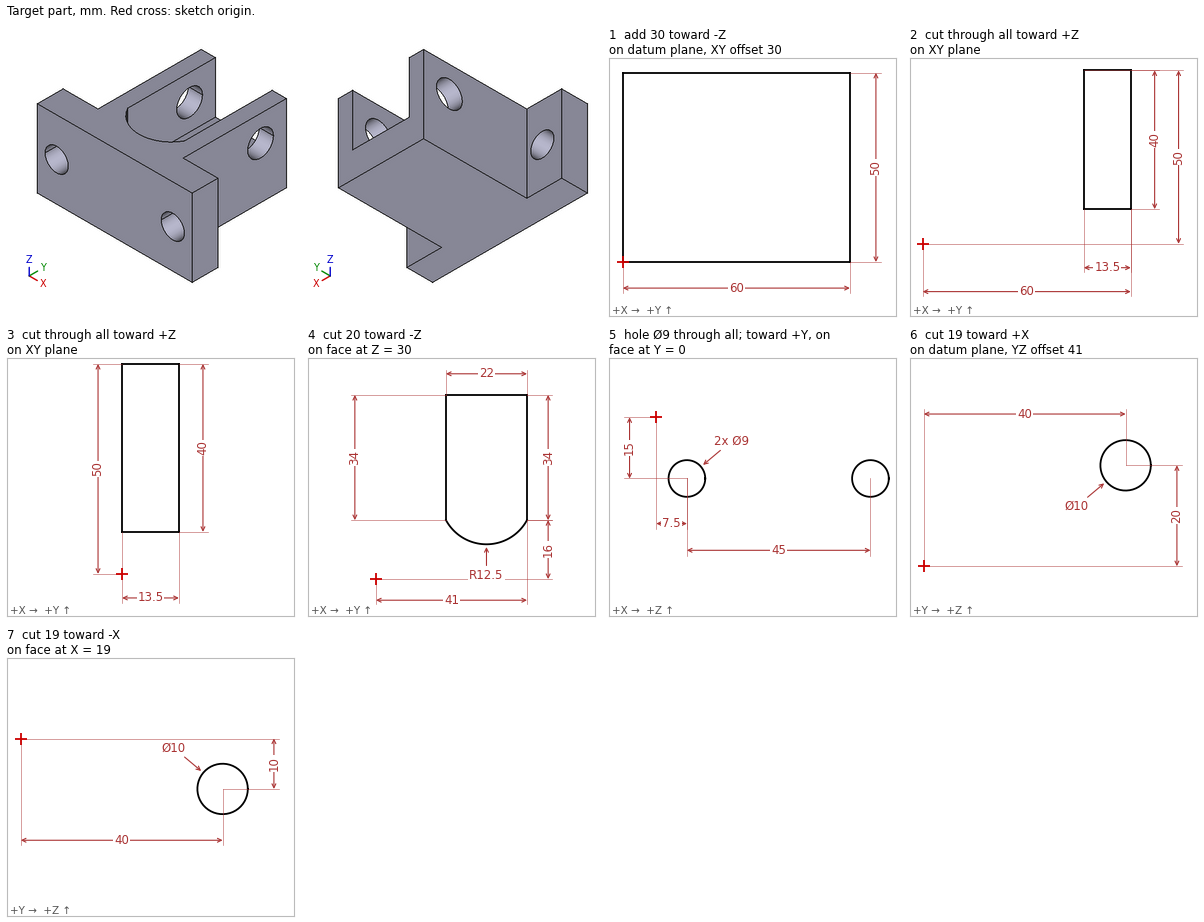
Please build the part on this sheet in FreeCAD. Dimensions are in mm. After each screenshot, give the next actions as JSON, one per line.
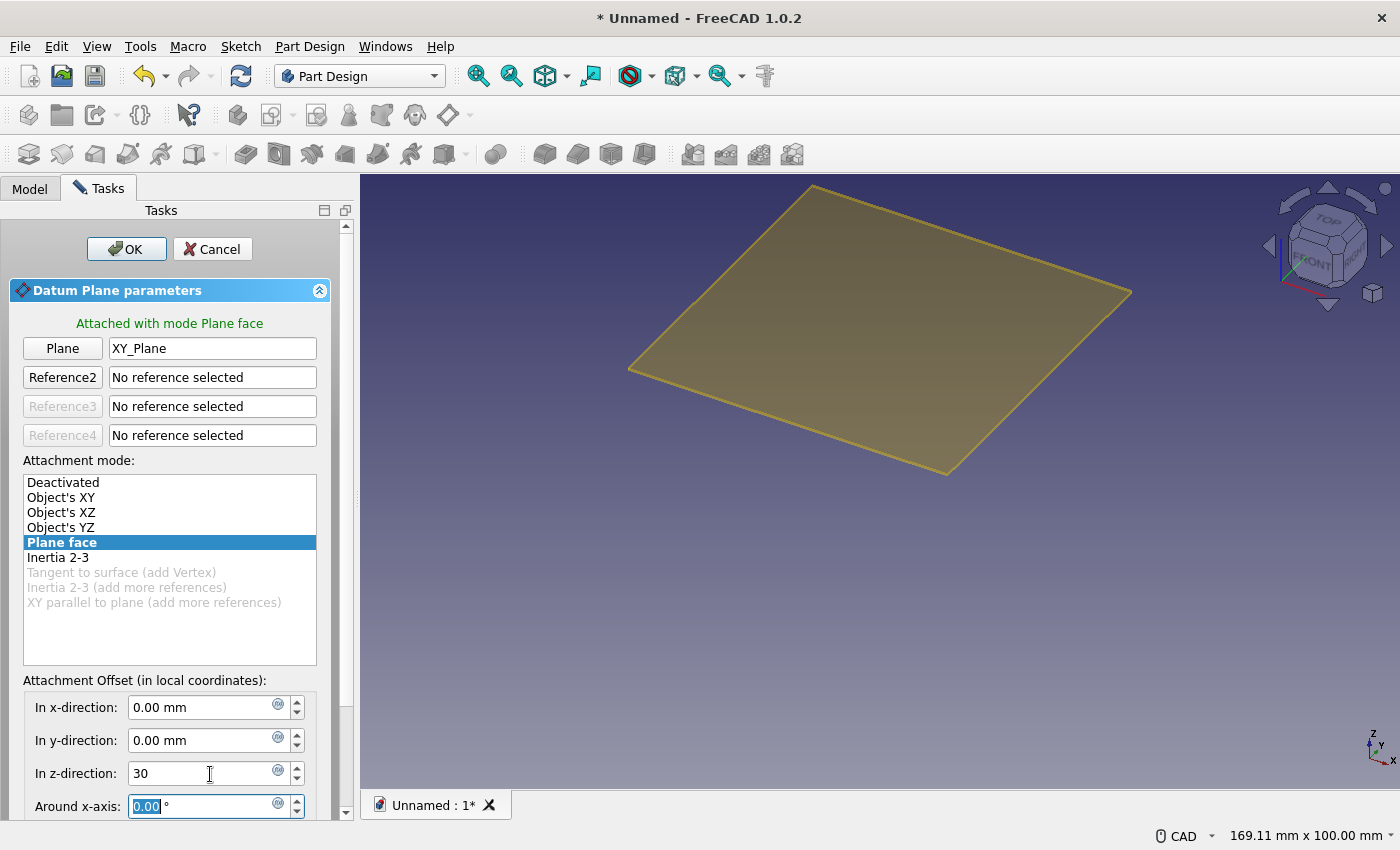
{"action": "left_click", "coordinate": [127, 249]}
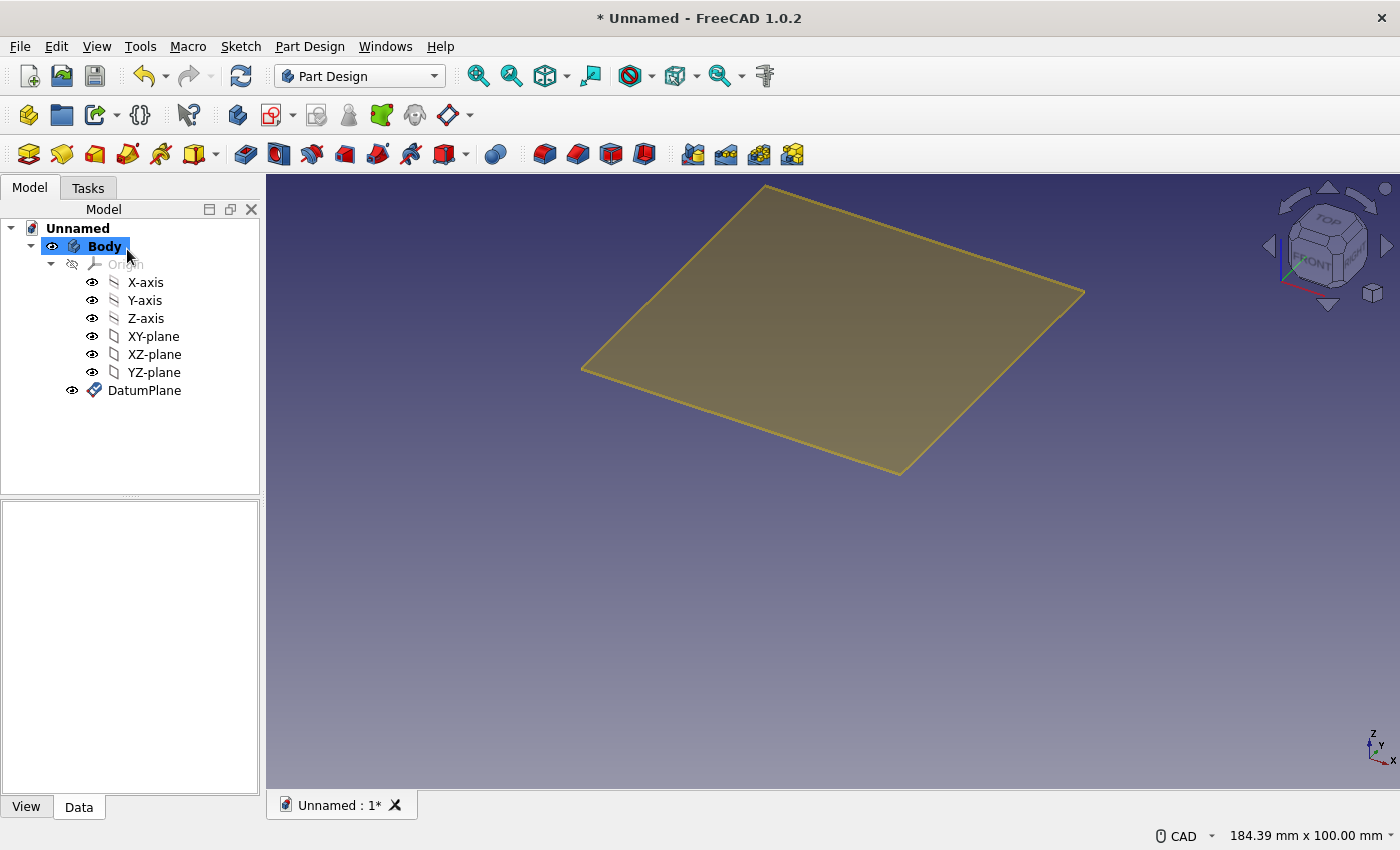
{"action": "left_click", "coordinate": [117, 390]}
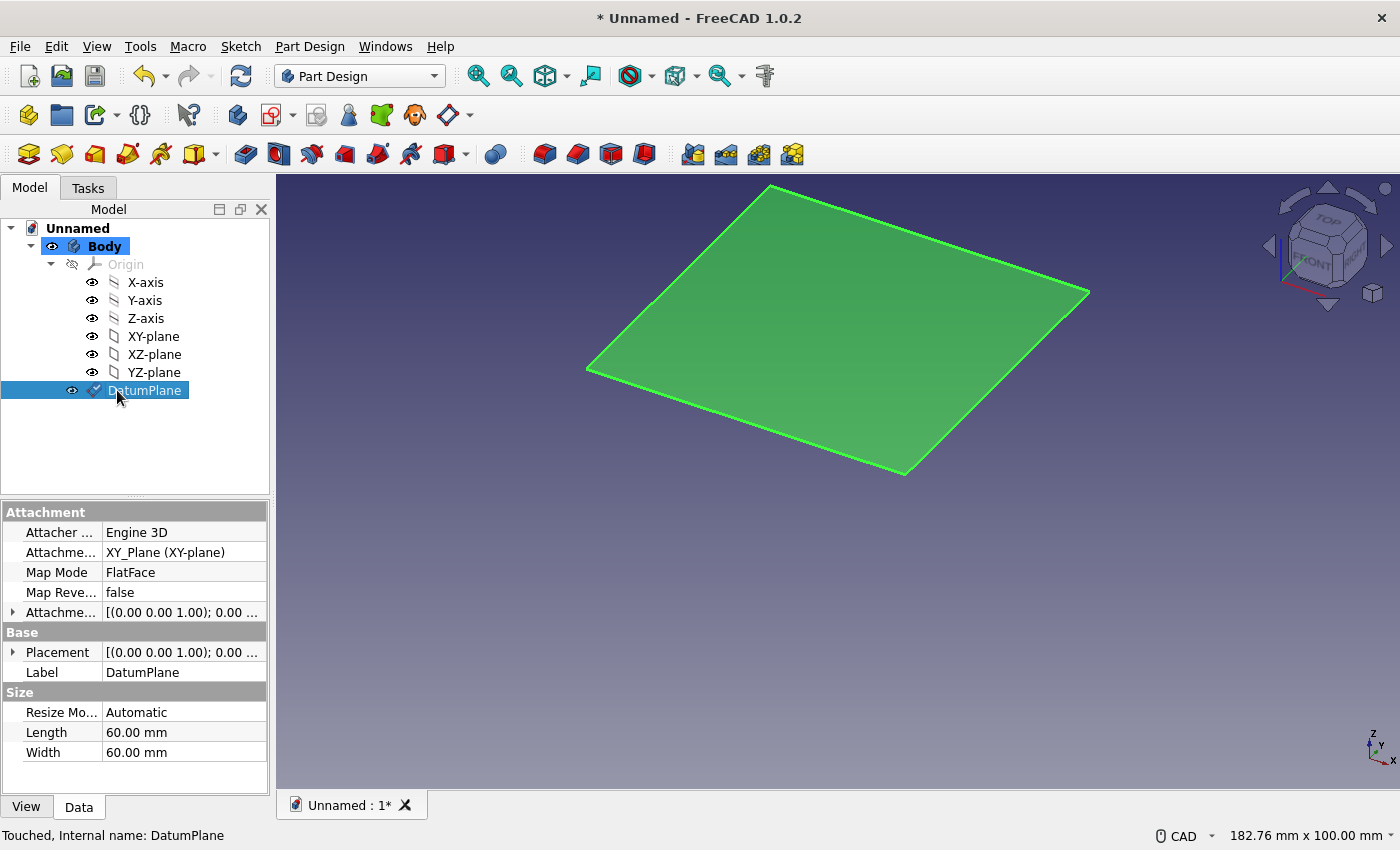
{"action": "left_click", "coordinate": [270, 116]}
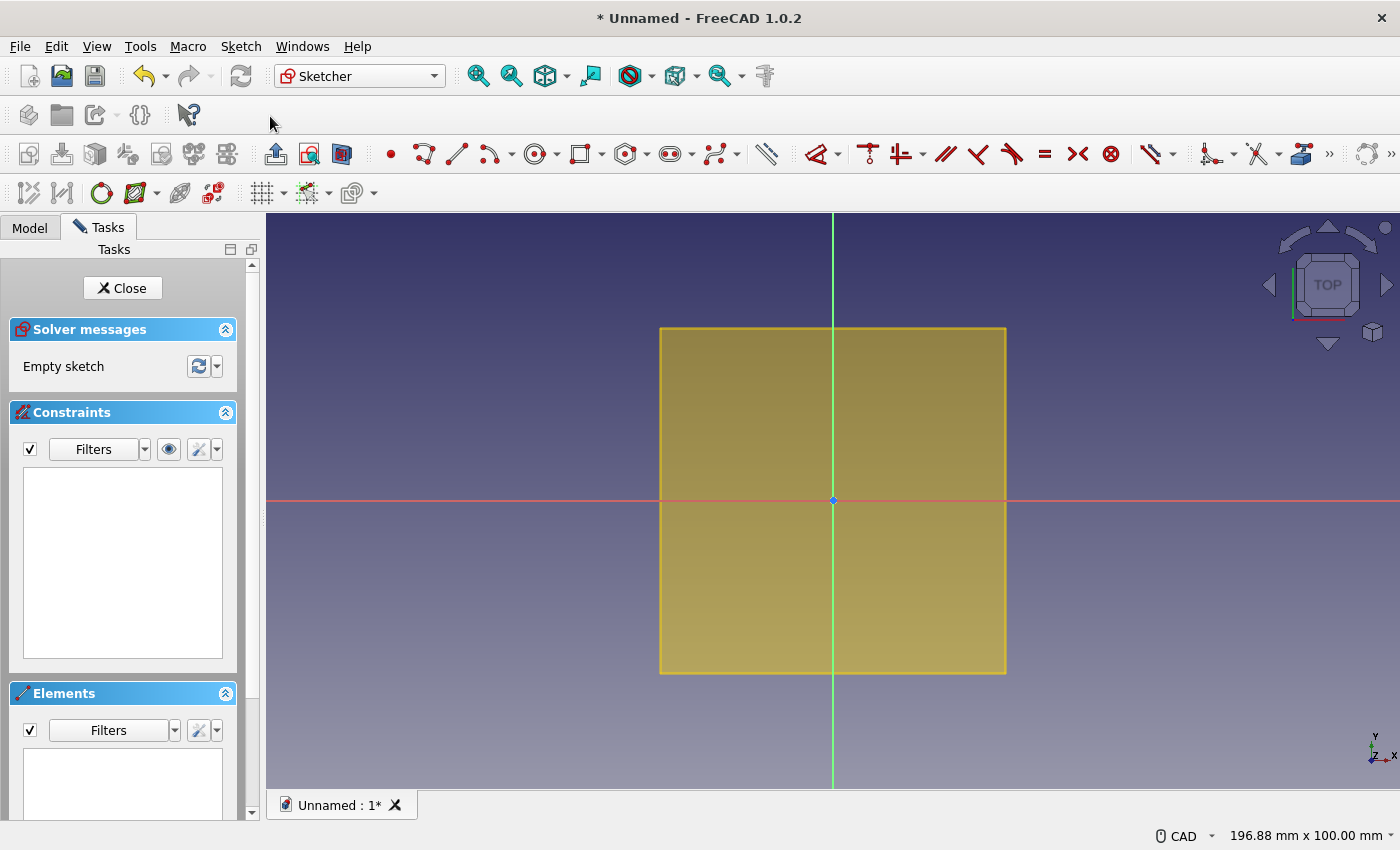
{"action": "scroll", "coordinate": [294, 761], "scroll_direction": "down", "scroll_amount": 1}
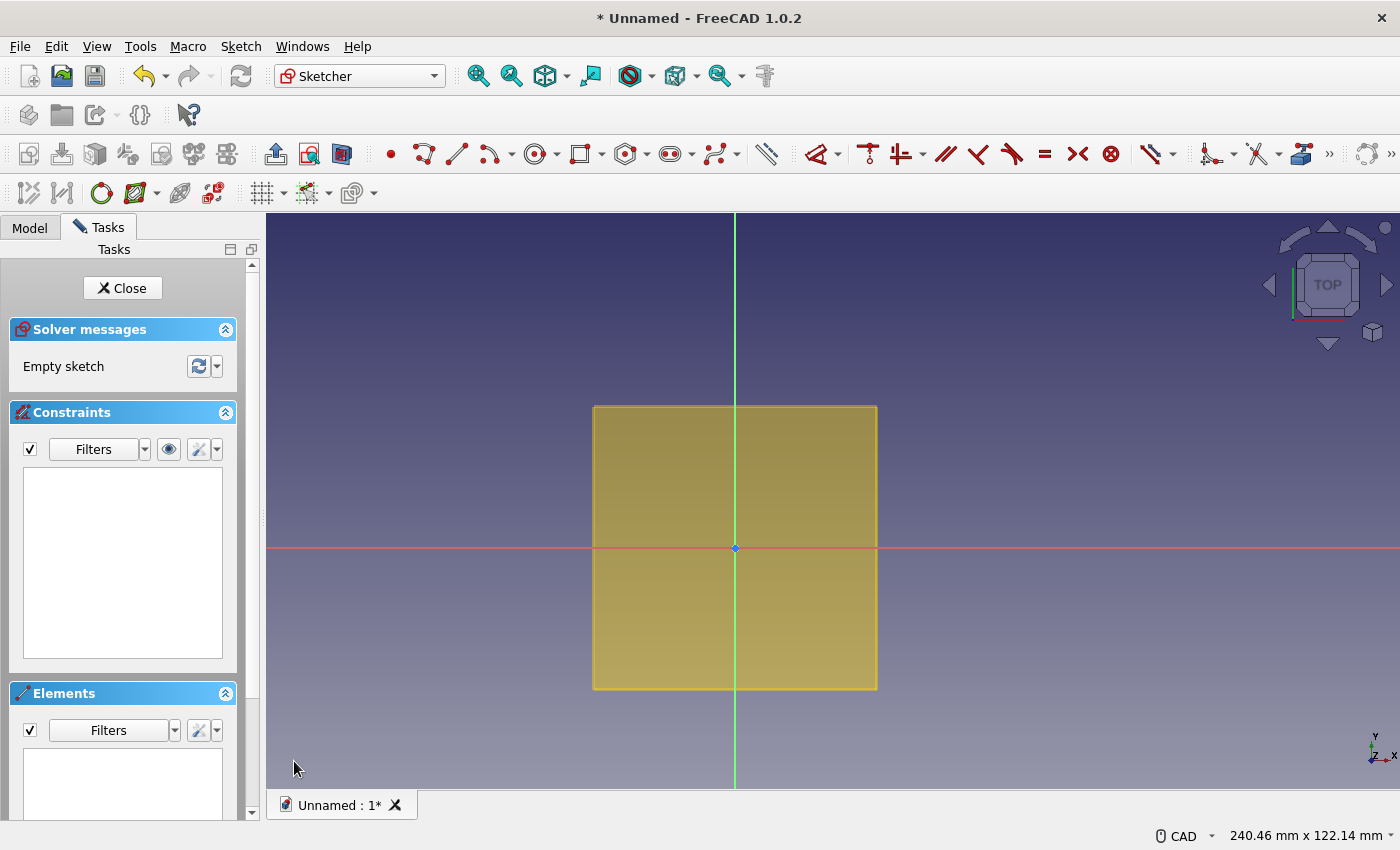
{"action": "scroll", "coordinate": [1105, 287], "scroll_direction": "up", "scroll_amount": 2}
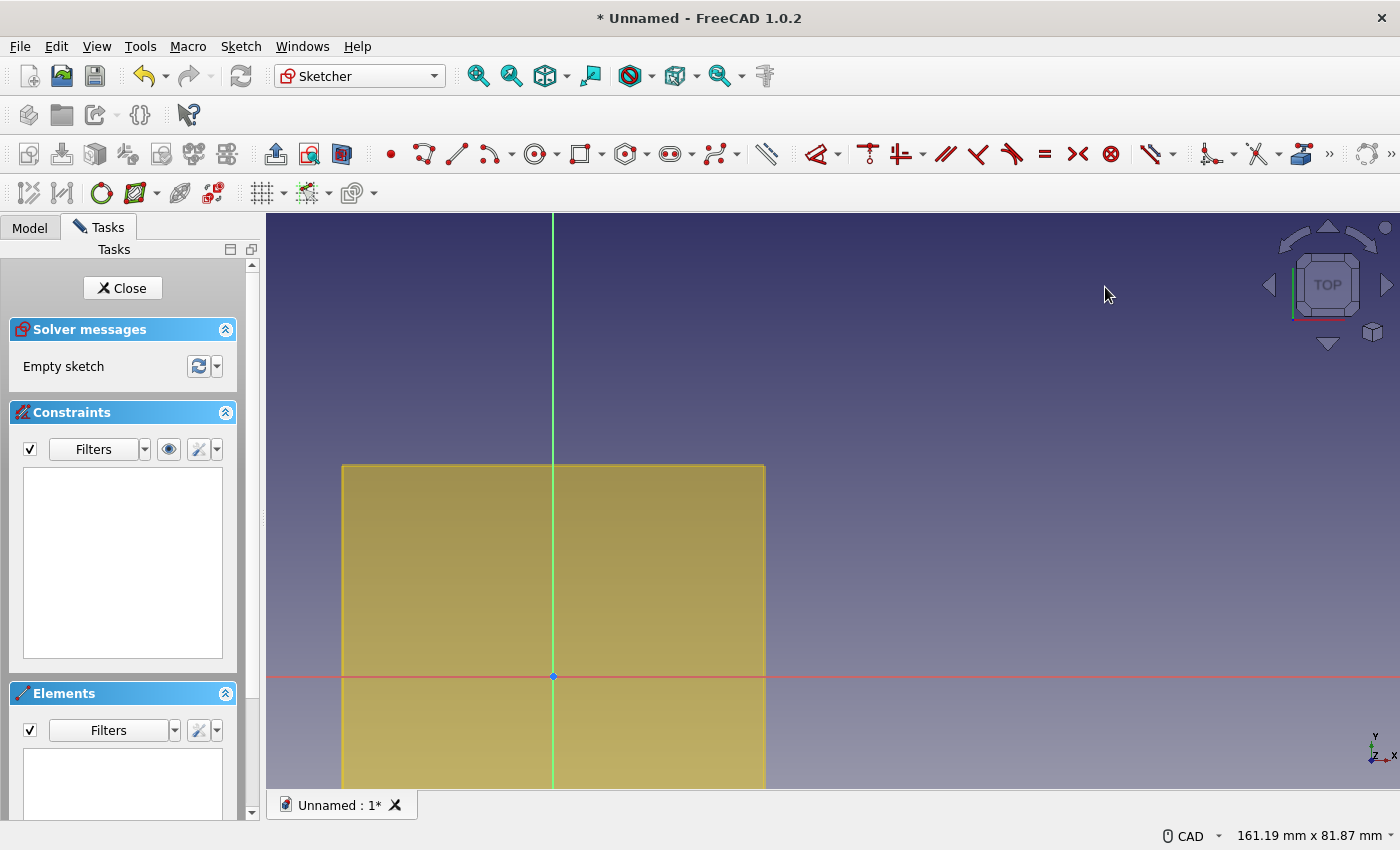
{"action": "key", "text": "g r"}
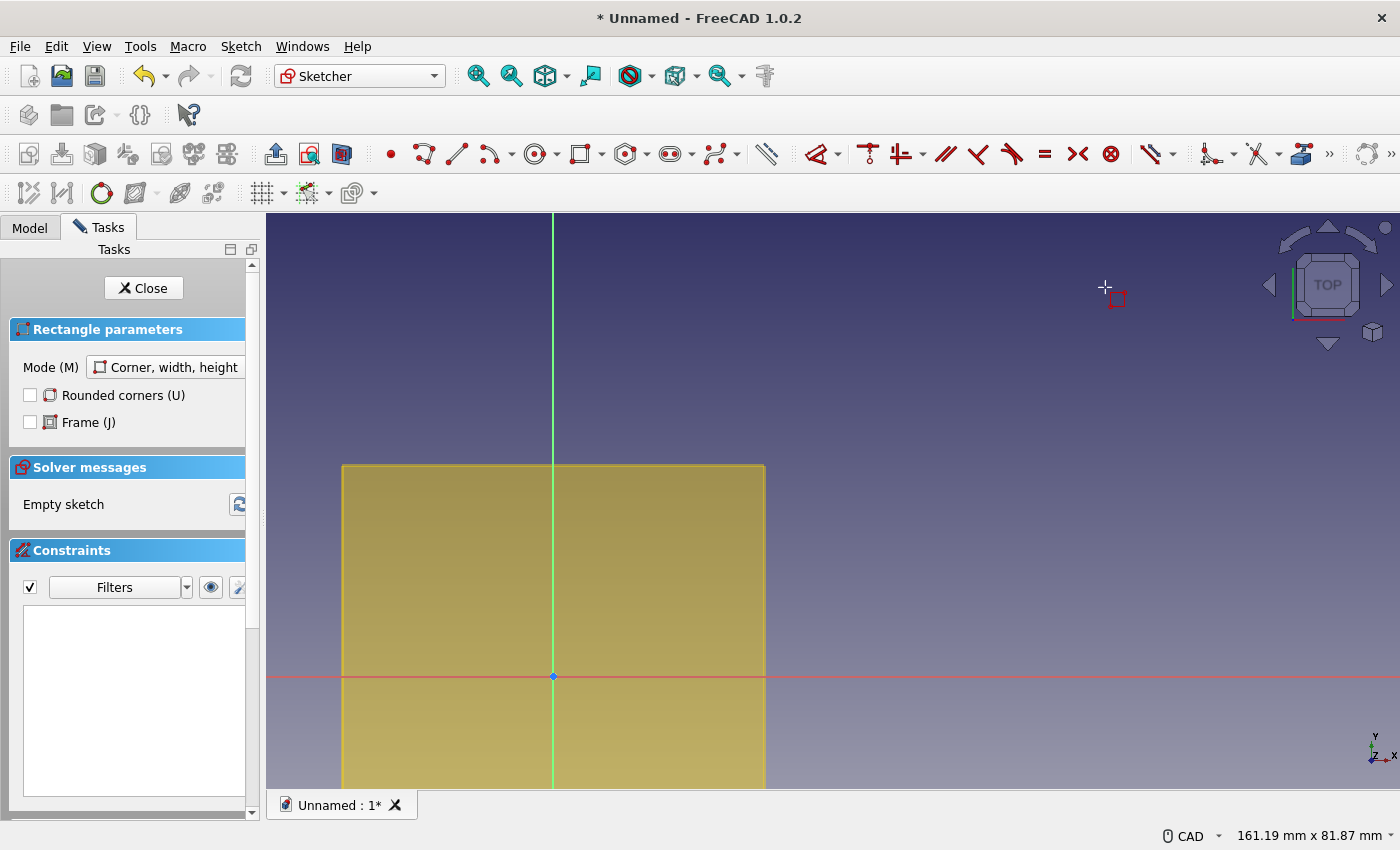
{"action": "left_click", "coordinate": [553, 677]}
{"action": "mouse_move", "coordinate": [975, 325]}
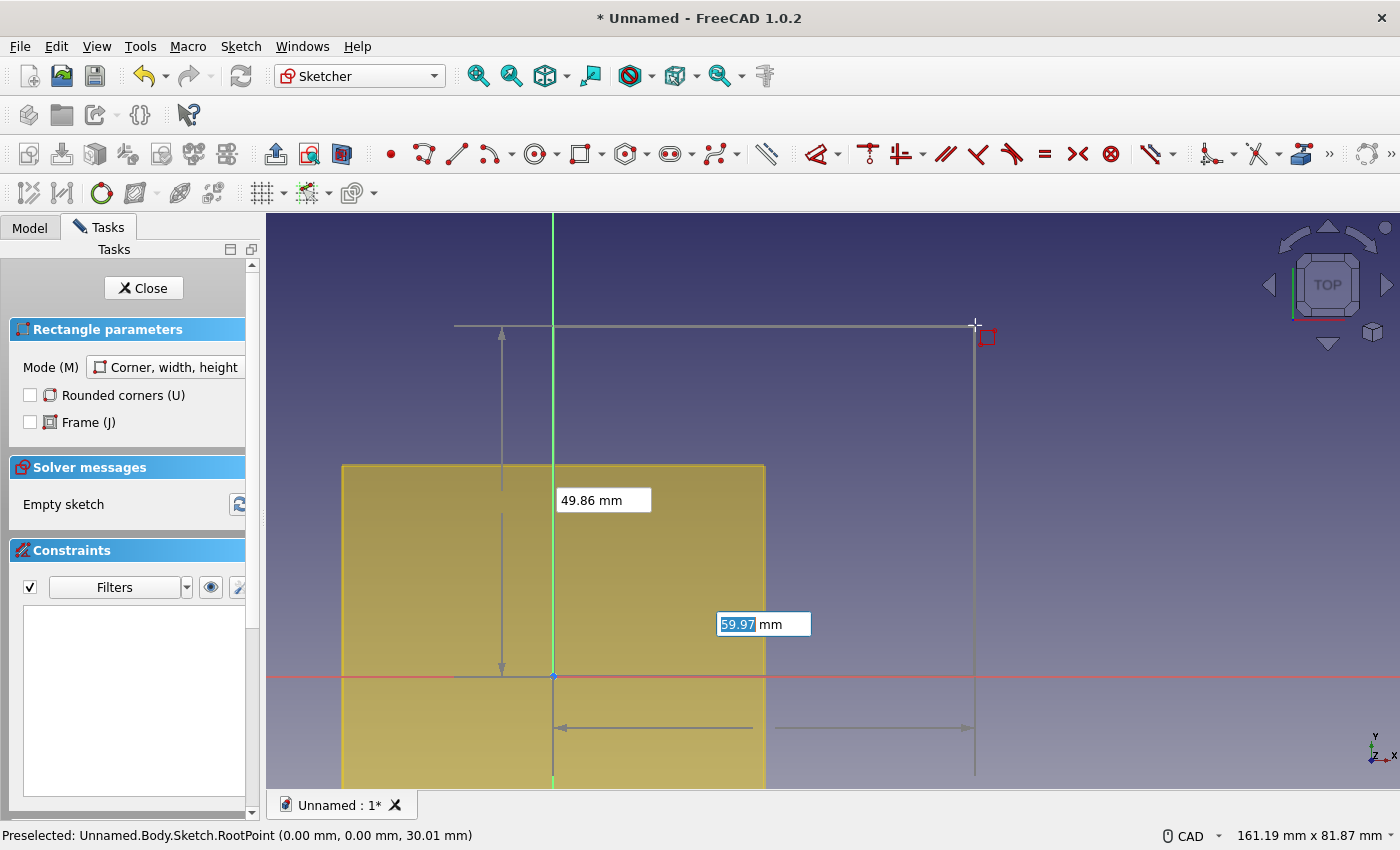
{"action": "type", "text": "60"}
{"action": "key", "text": "Tab"}
{"action": "type", "text": "50"}
{"action": "key", "text": "Return"}
{"action": "key", "text": "Escape"}